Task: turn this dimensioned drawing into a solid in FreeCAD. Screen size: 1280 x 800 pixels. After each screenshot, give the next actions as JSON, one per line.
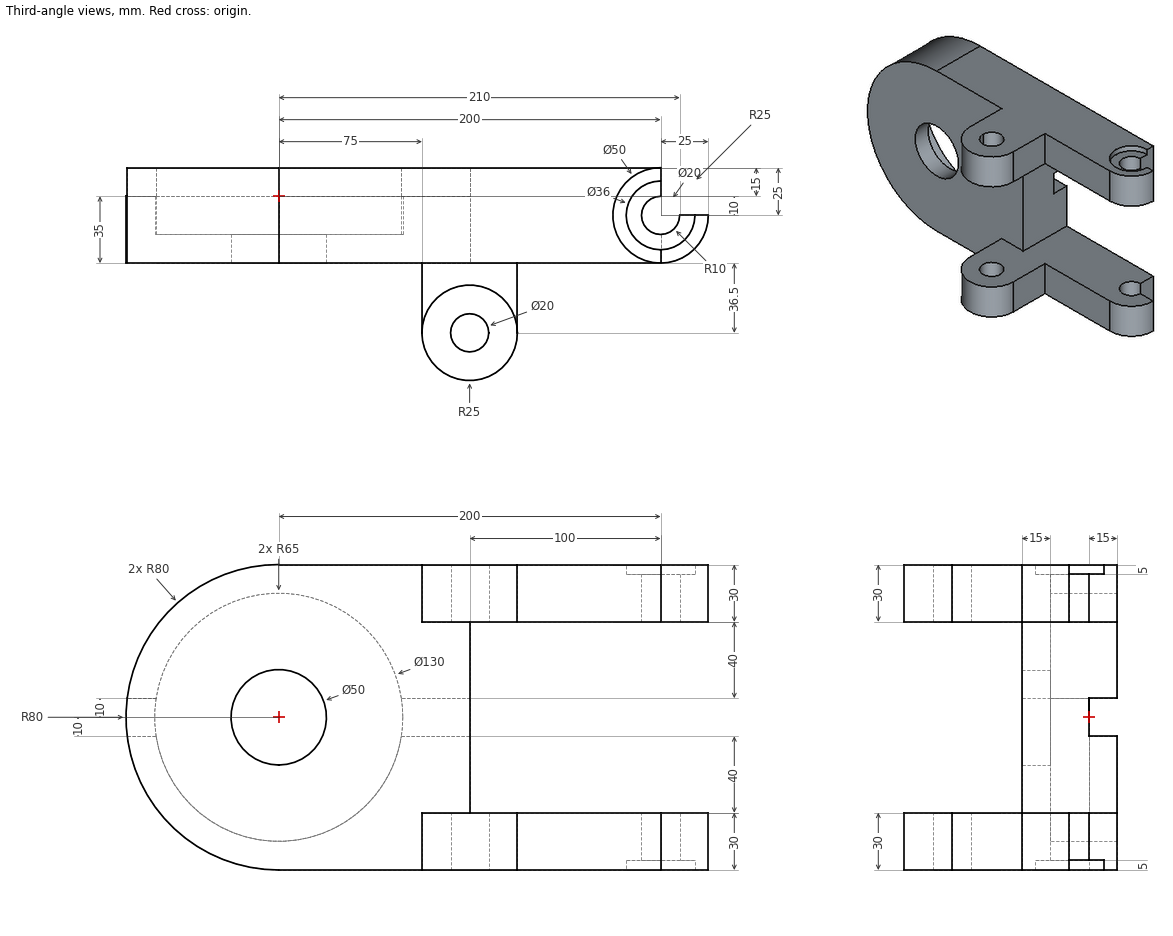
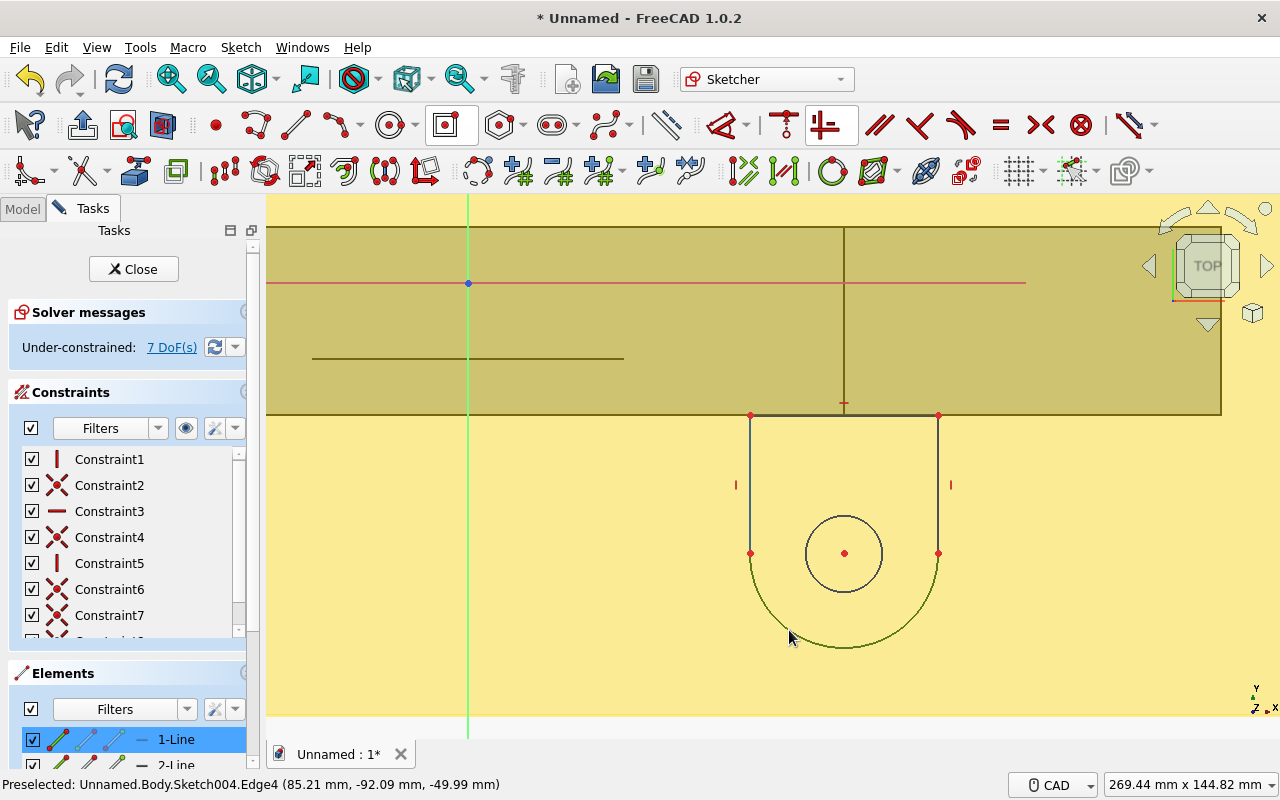
{"action": "left_click", "coordinate": [962, 126]}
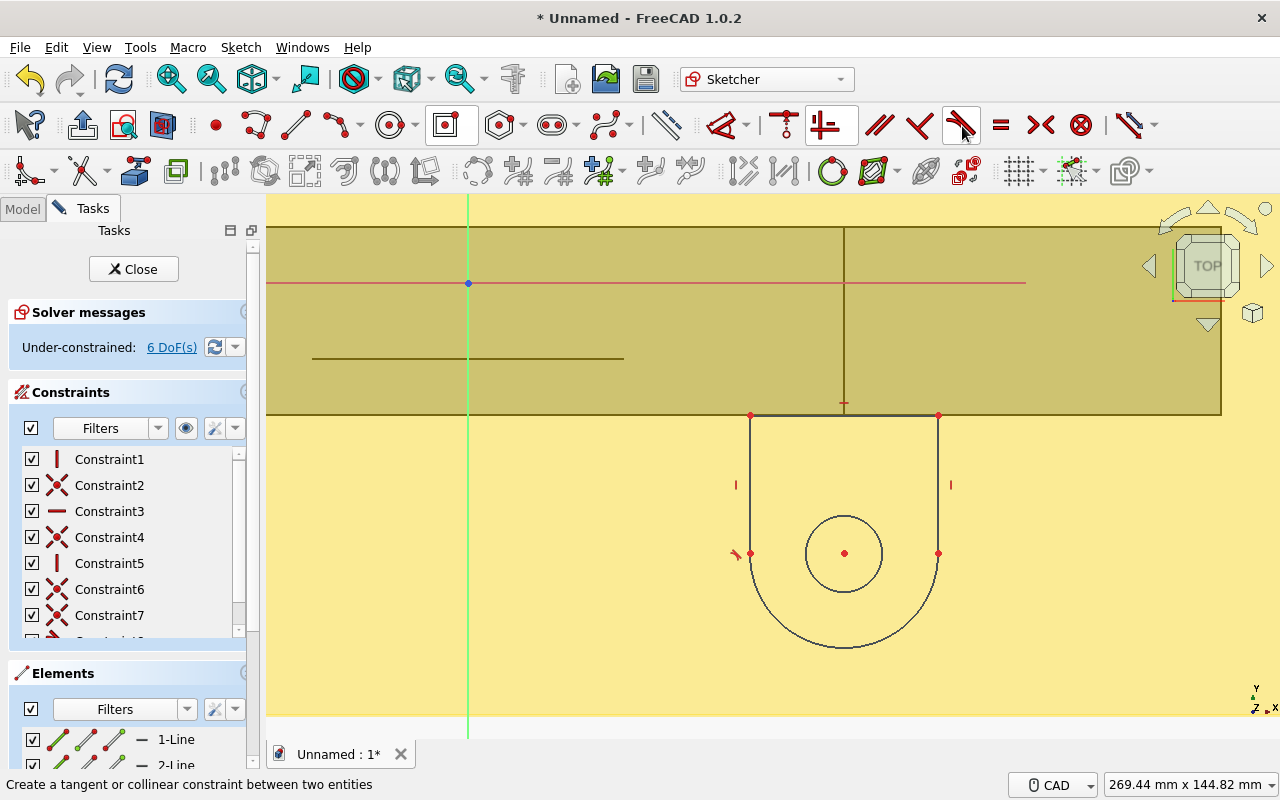
{"action": "left_click", "coordinate": [938, 457]}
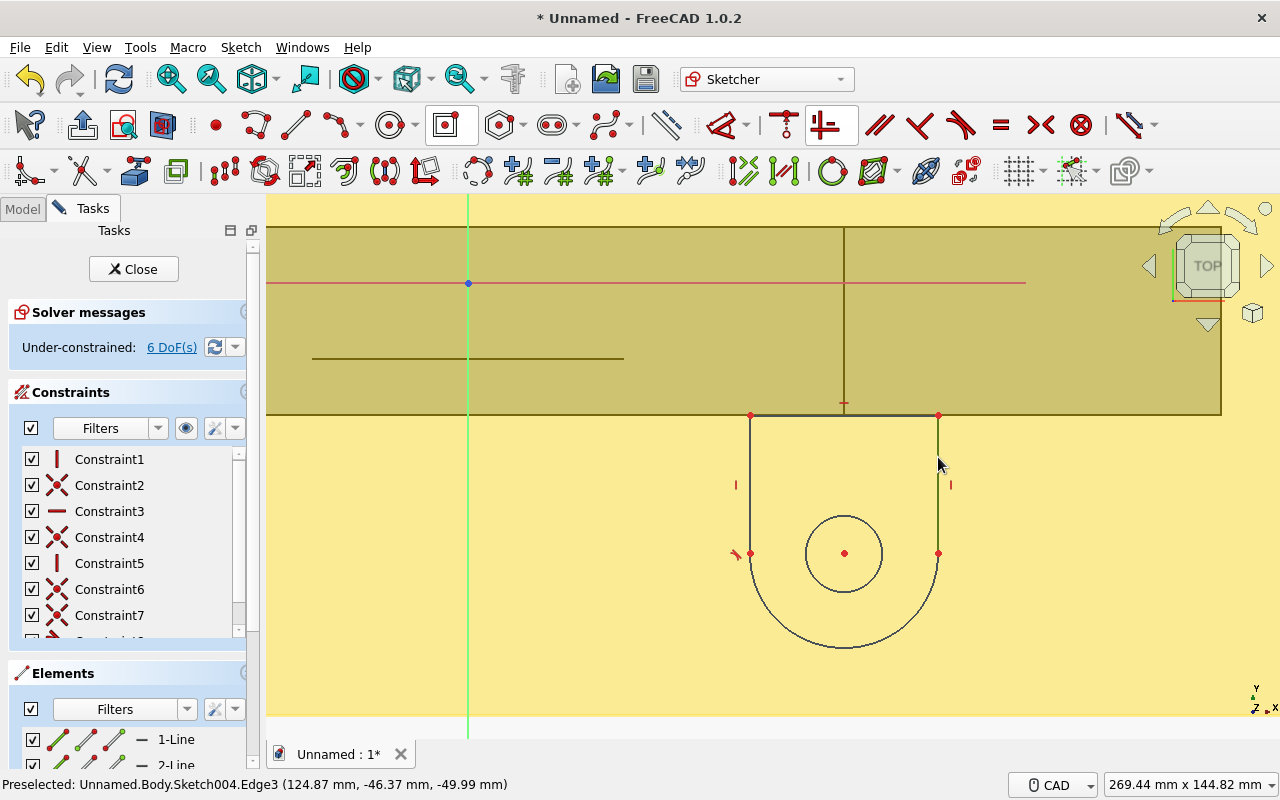
{"action": "left_click", "coordinate": [789, 630]}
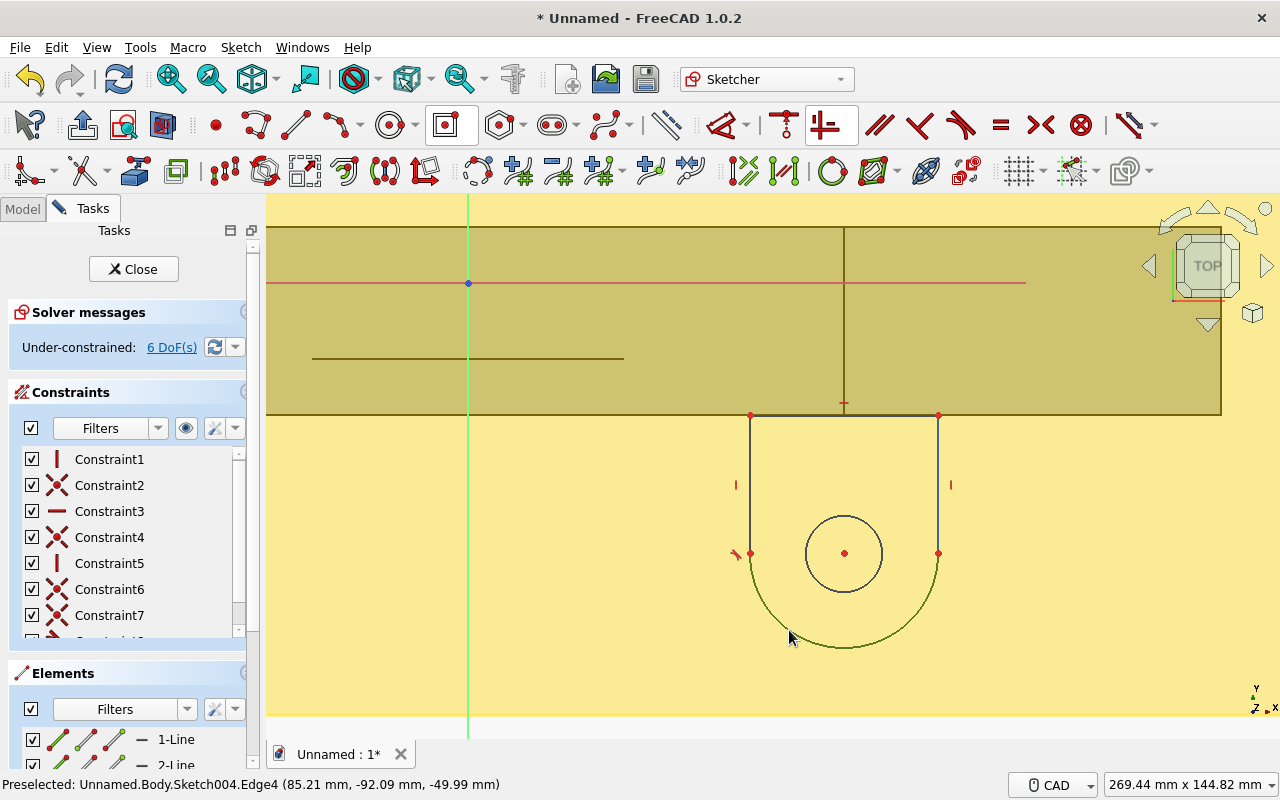
{"action": "left_click", "coordinate": [962, 126]}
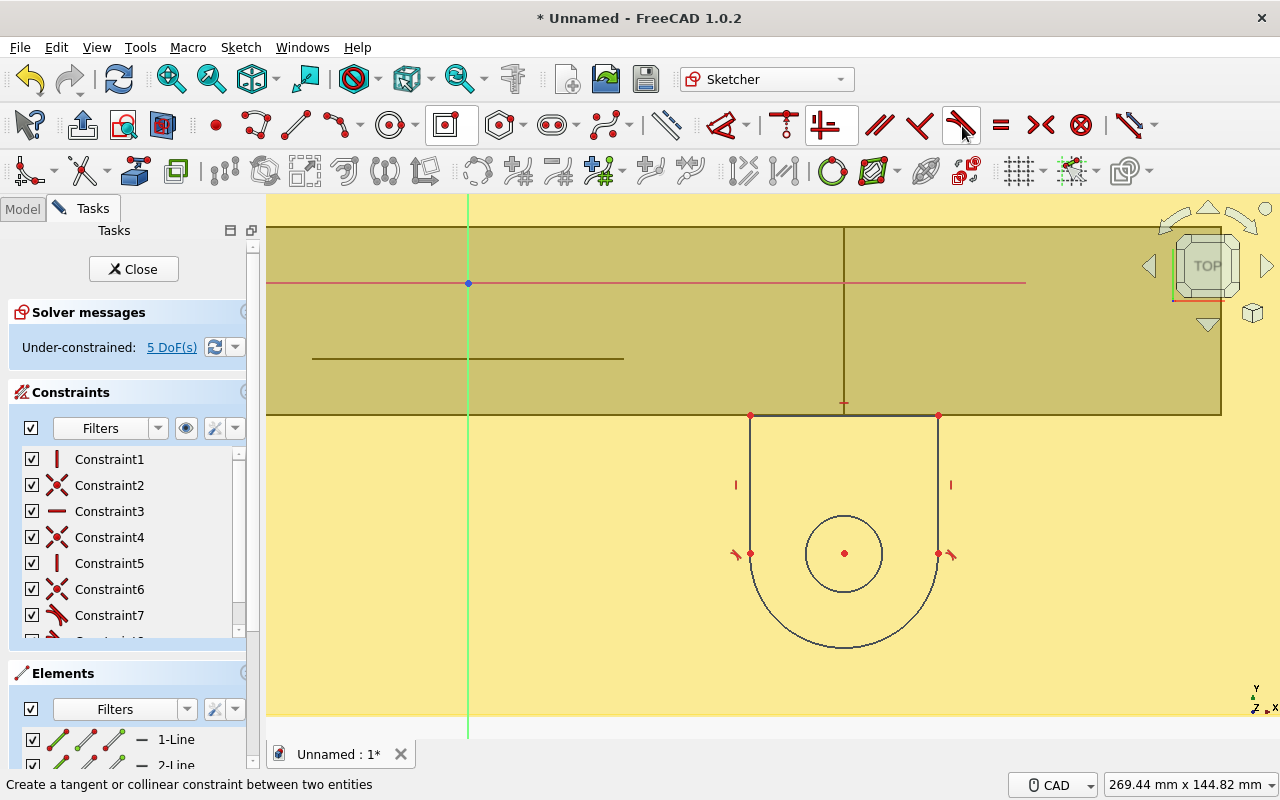
{"action": "left_click", "coordinate": [722, 126]}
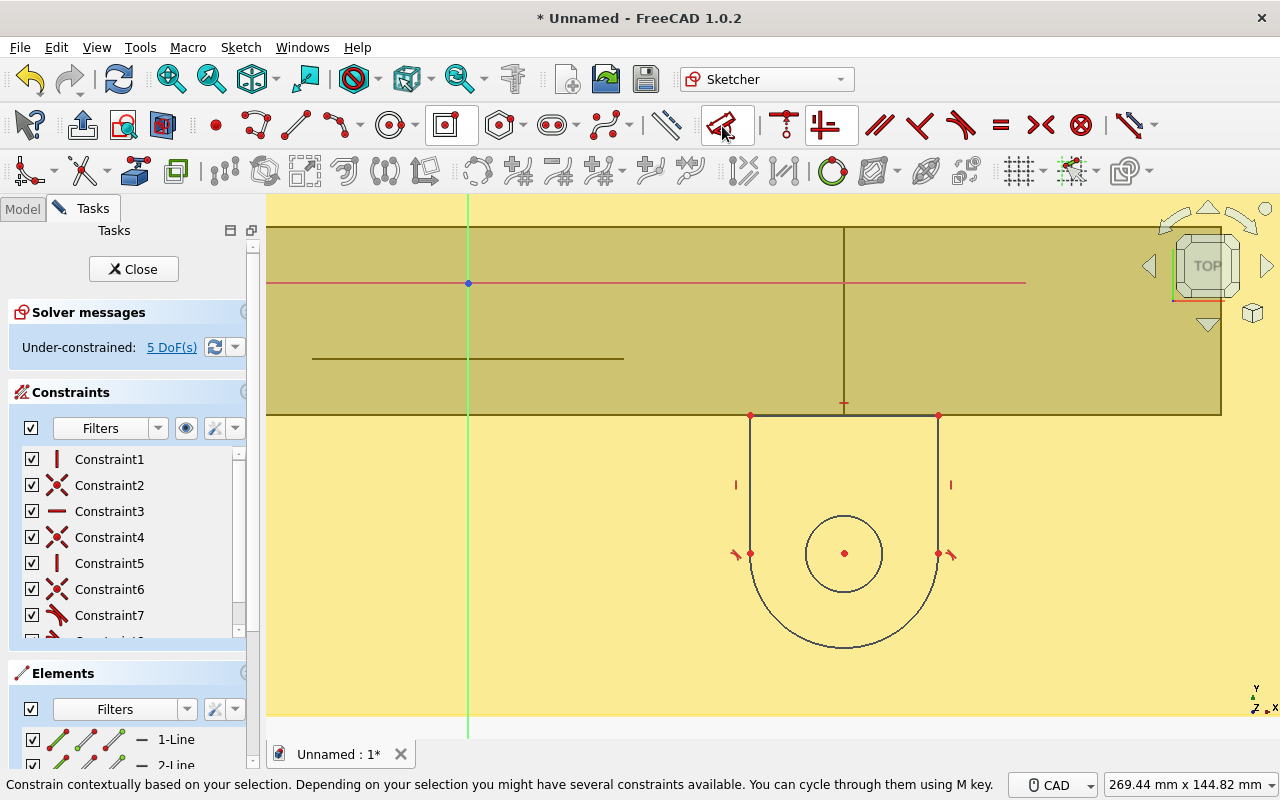
{"action": "left_click", "coordinate": [789, 630]}
{"action": "left_click", "coordinate": [770, 656]}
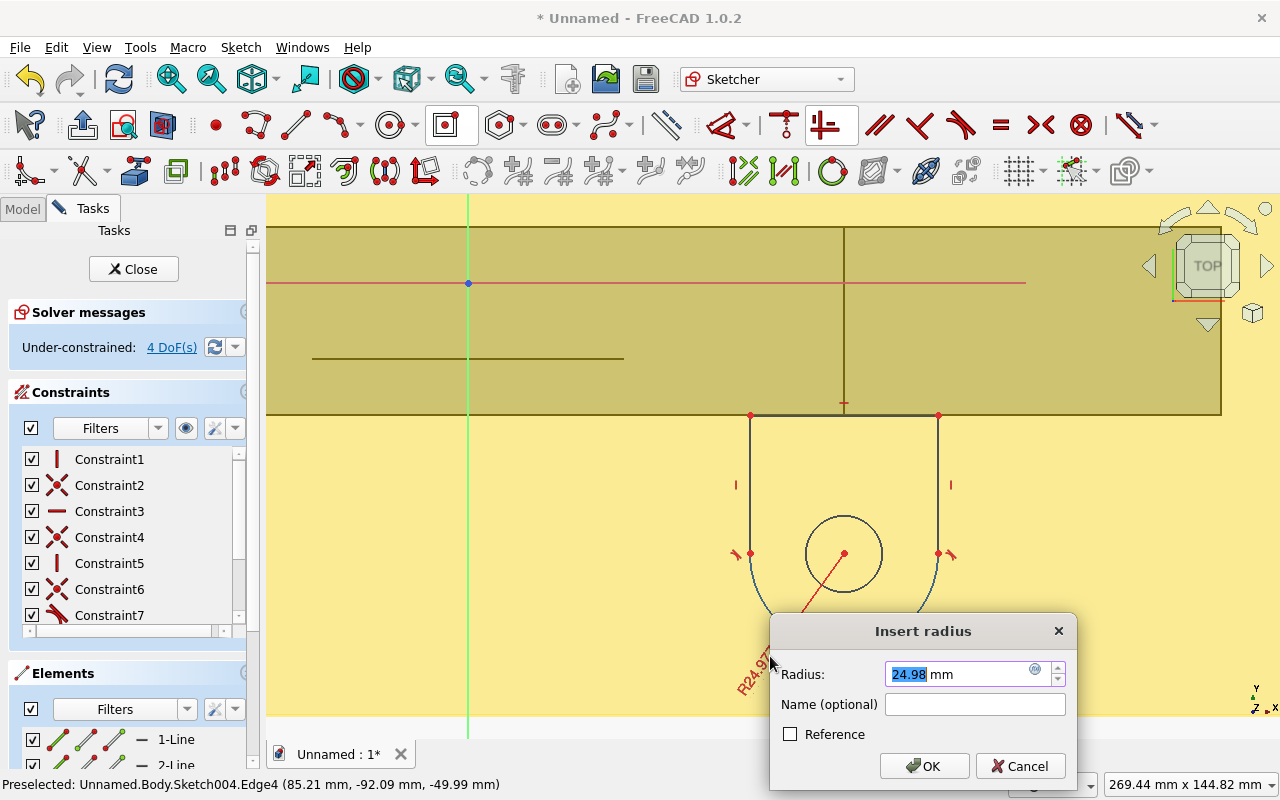
{"action": "type", "text": "25"}
{"action": "key", "text": "Return"}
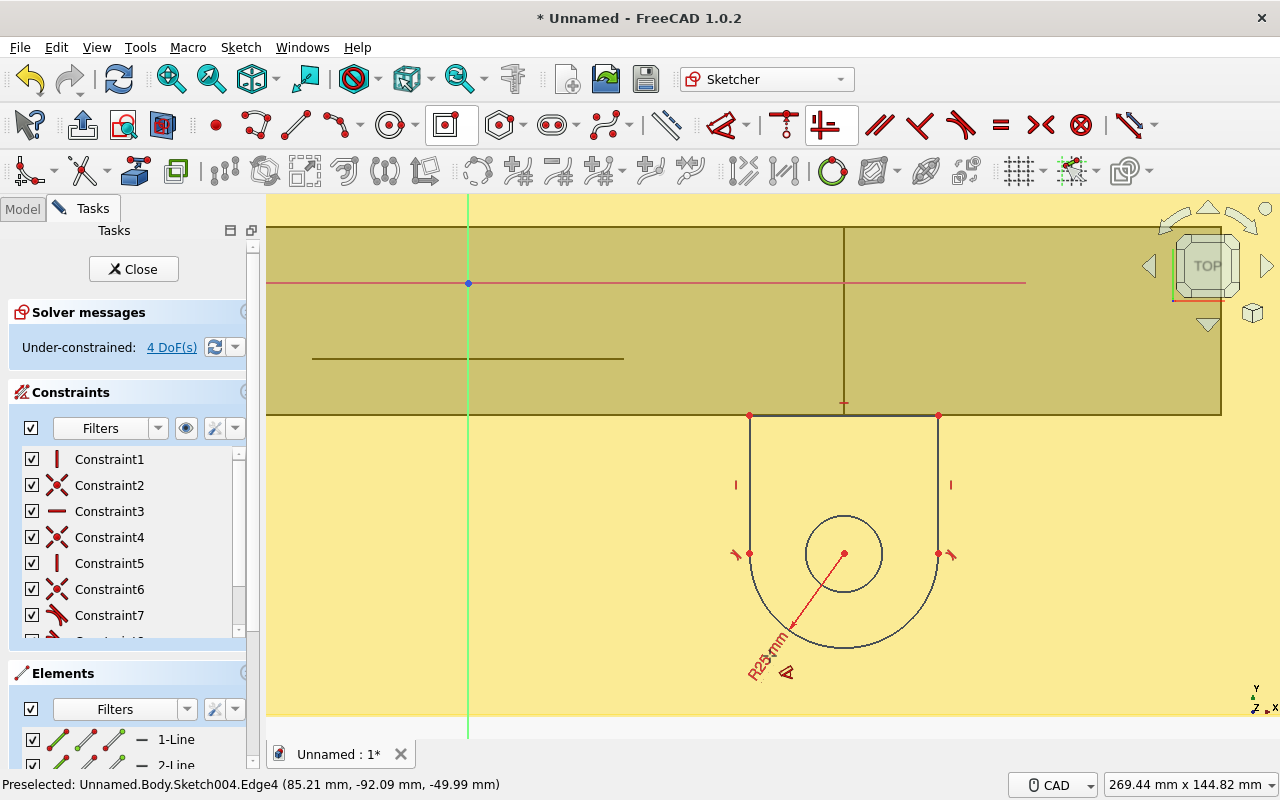
{"action": "left_click", "coordinate": [871, 527]}
{"action": "left_click", "coordinate": [894, 504]}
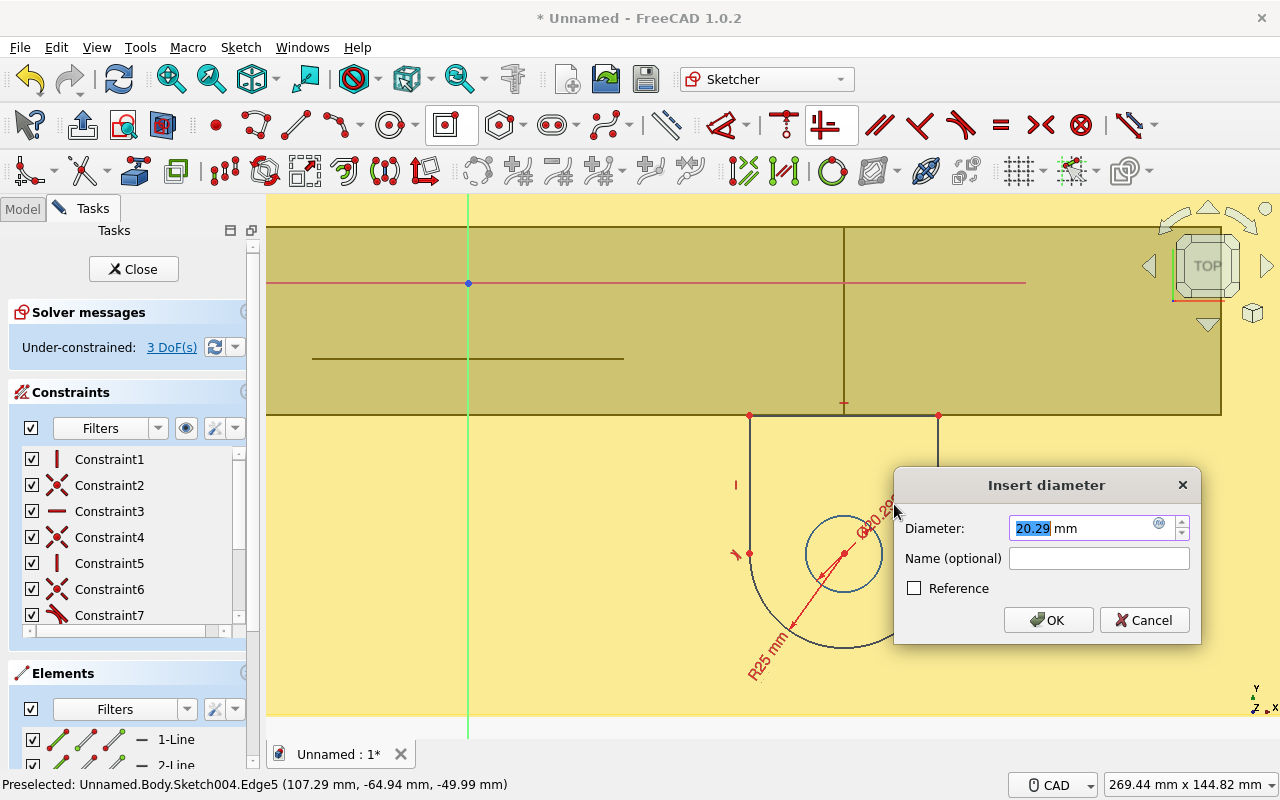
{"action": "type", "text": "20"}
{"action": "key", "text": "Return"}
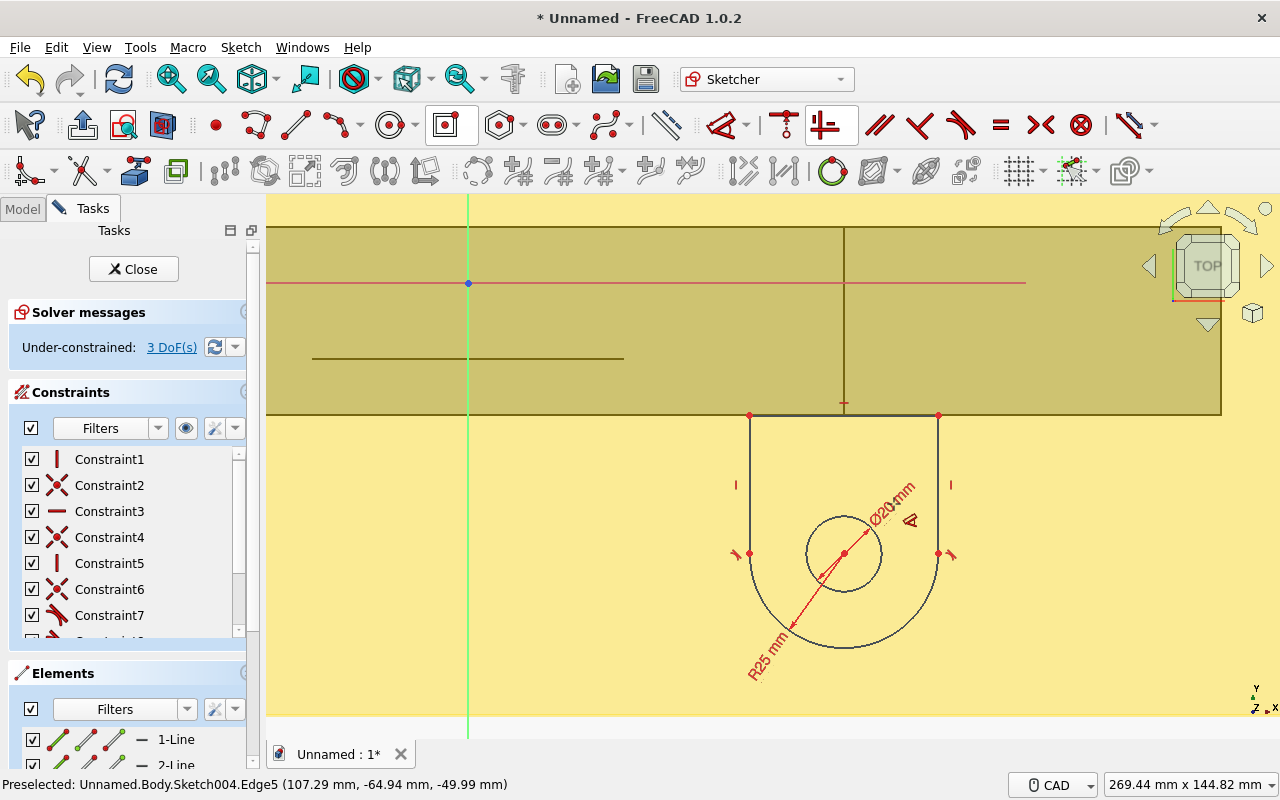
{"action": "left_click", "coordinate": [750, 554]}
{"action": "left_click", "coordinate": [609, 249]}